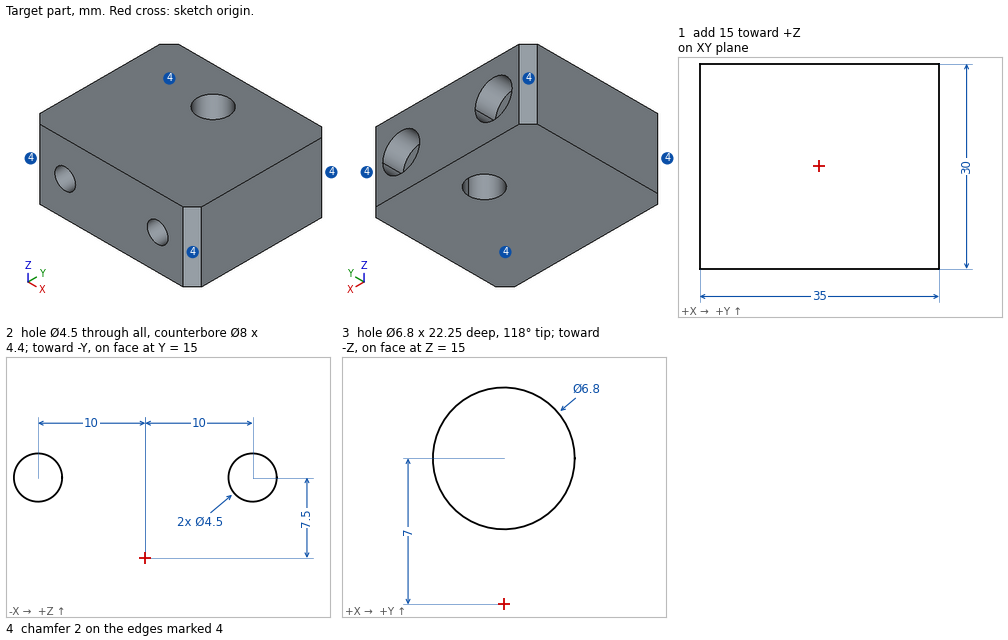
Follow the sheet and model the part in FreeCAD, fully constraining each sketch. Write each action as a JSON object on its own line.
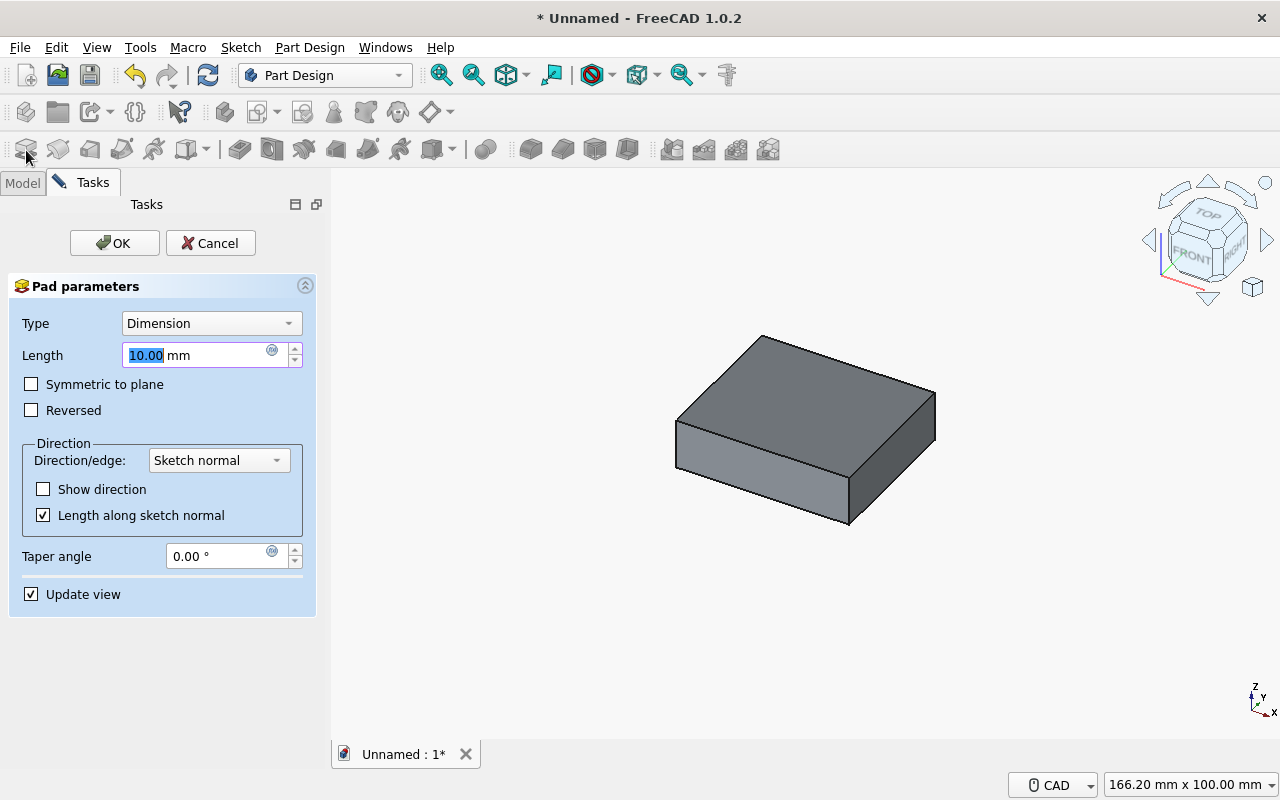
{"action": "type", "text": "15"}
{"action": "key", "text": "Tab"}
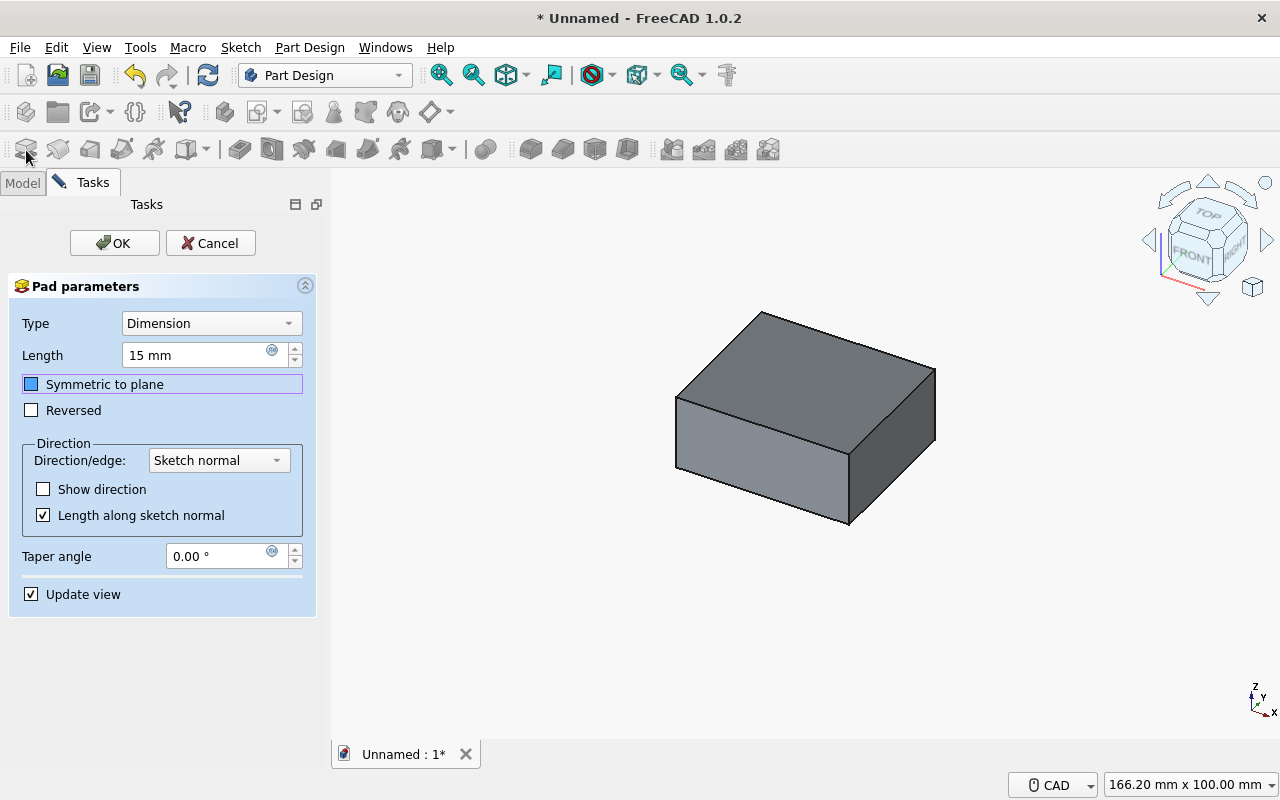
{"action": "left_click", "coordinate": [115, 243]}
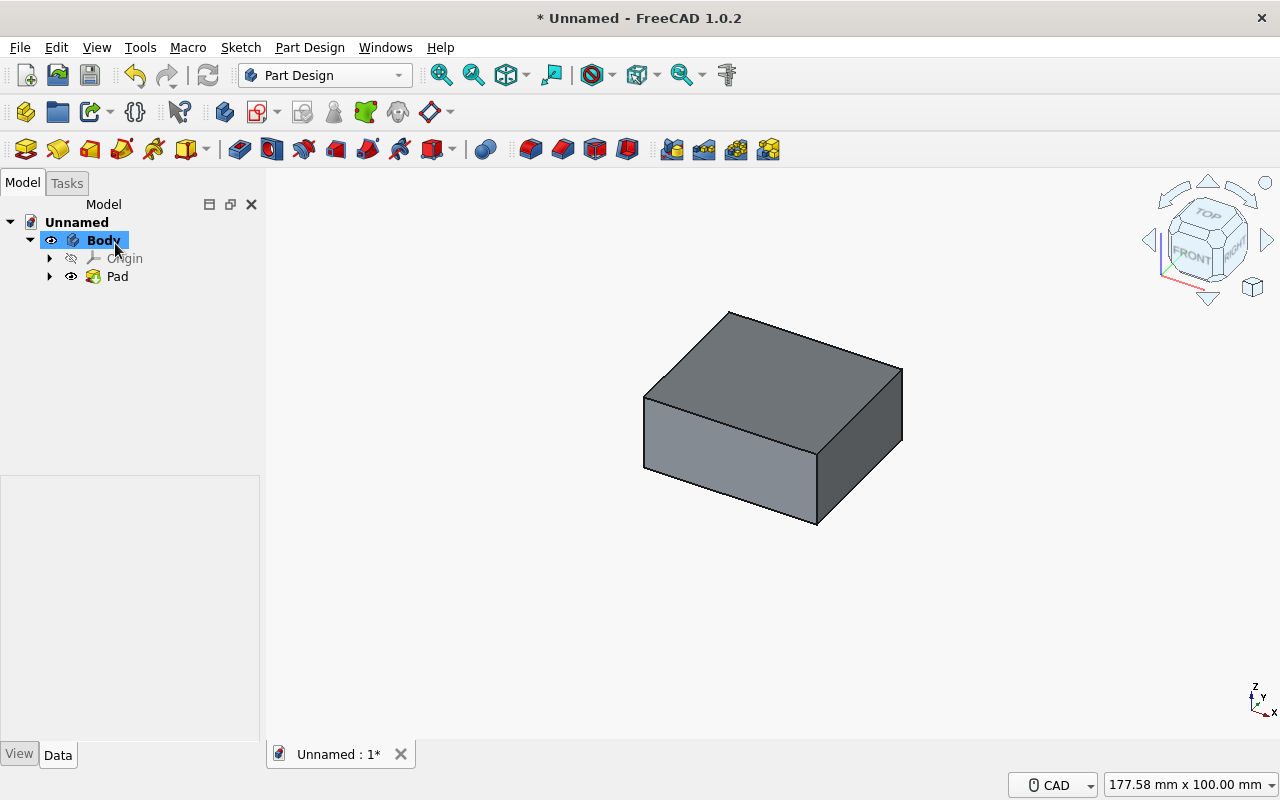
{"action": "left_click", "coordinate": [442, 76]}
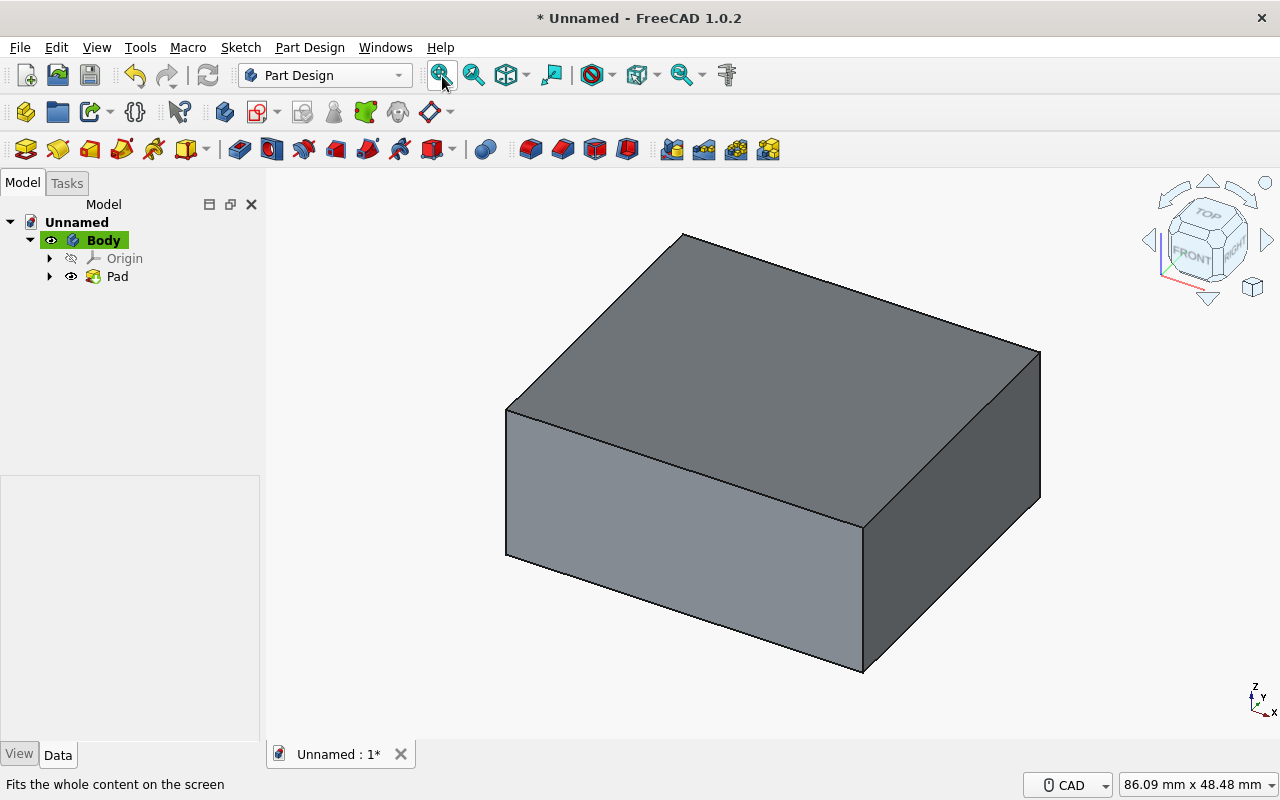
{"action": "key", "text": "4"}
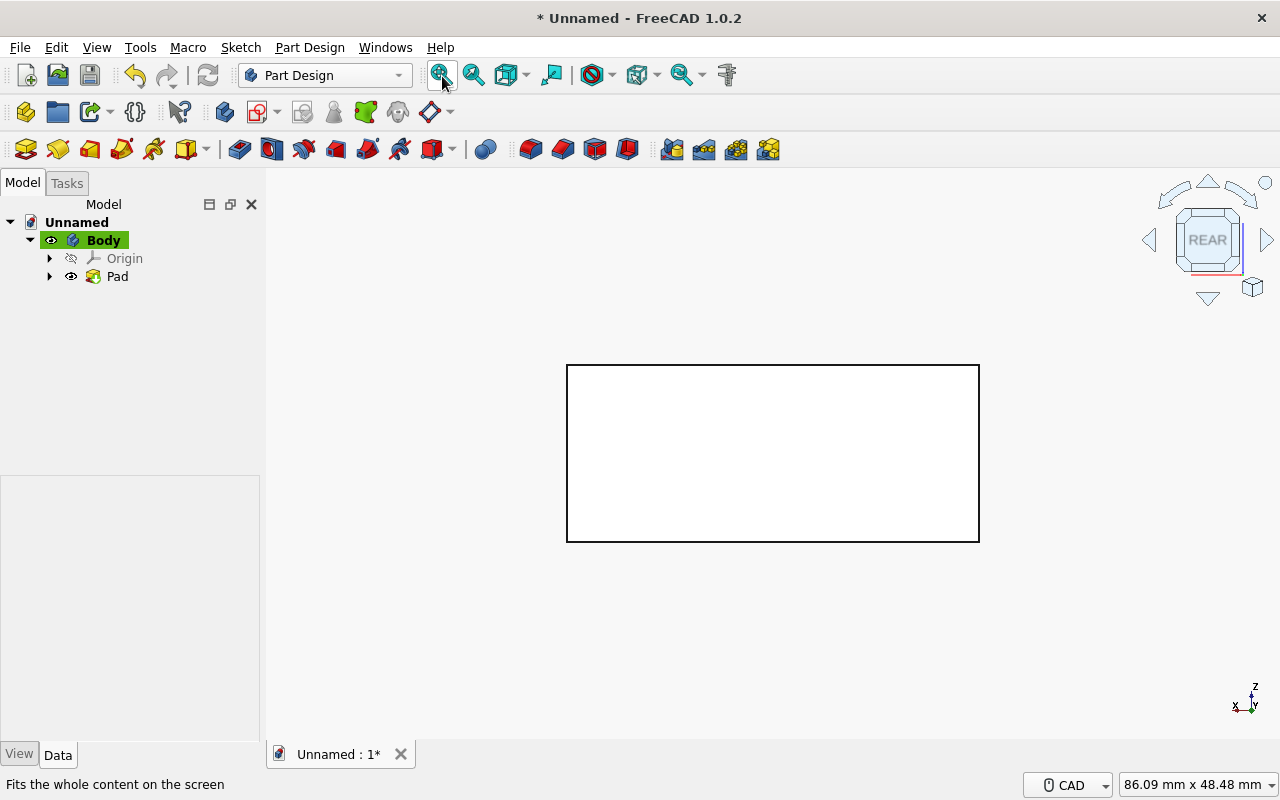
{"action": "key", "text": "v f"}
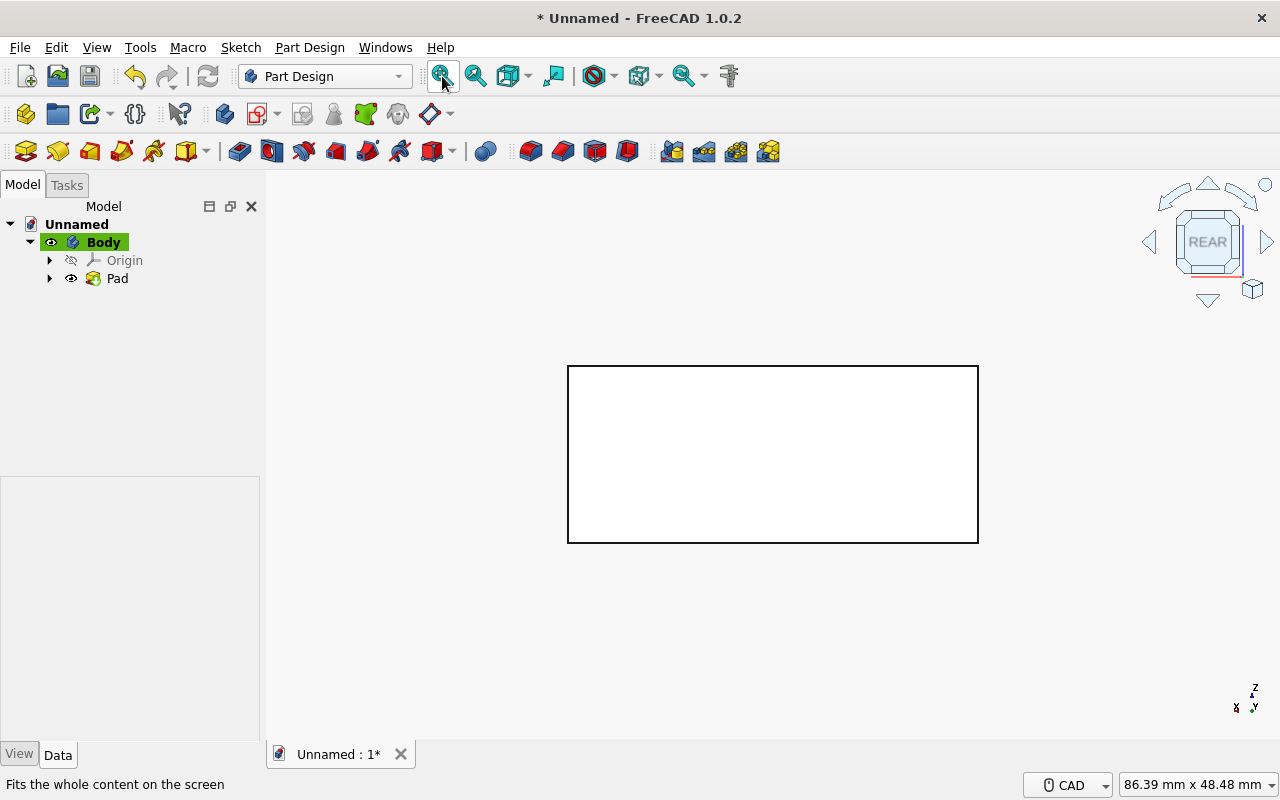
{"action": "left_click", "coordinate": [656, 454]}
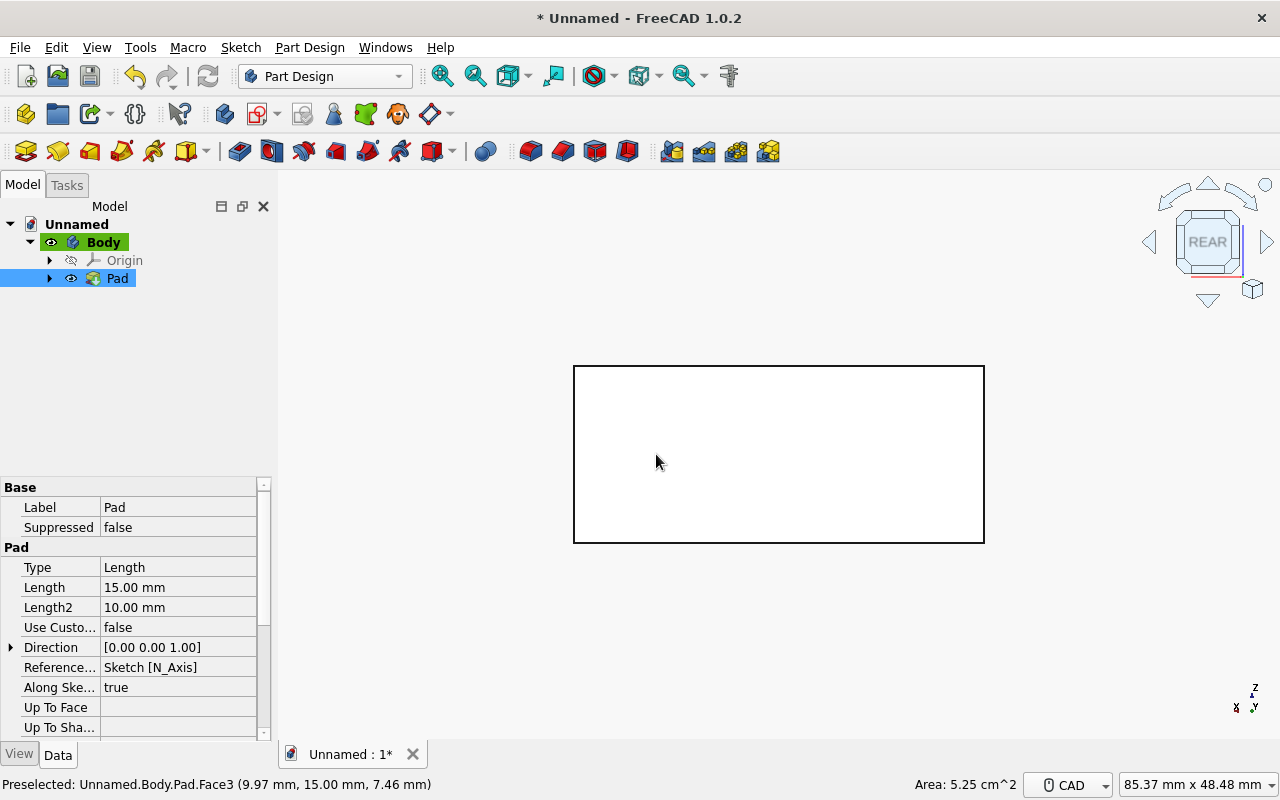
{"action": "left_click", "coordinate": [258, 114]}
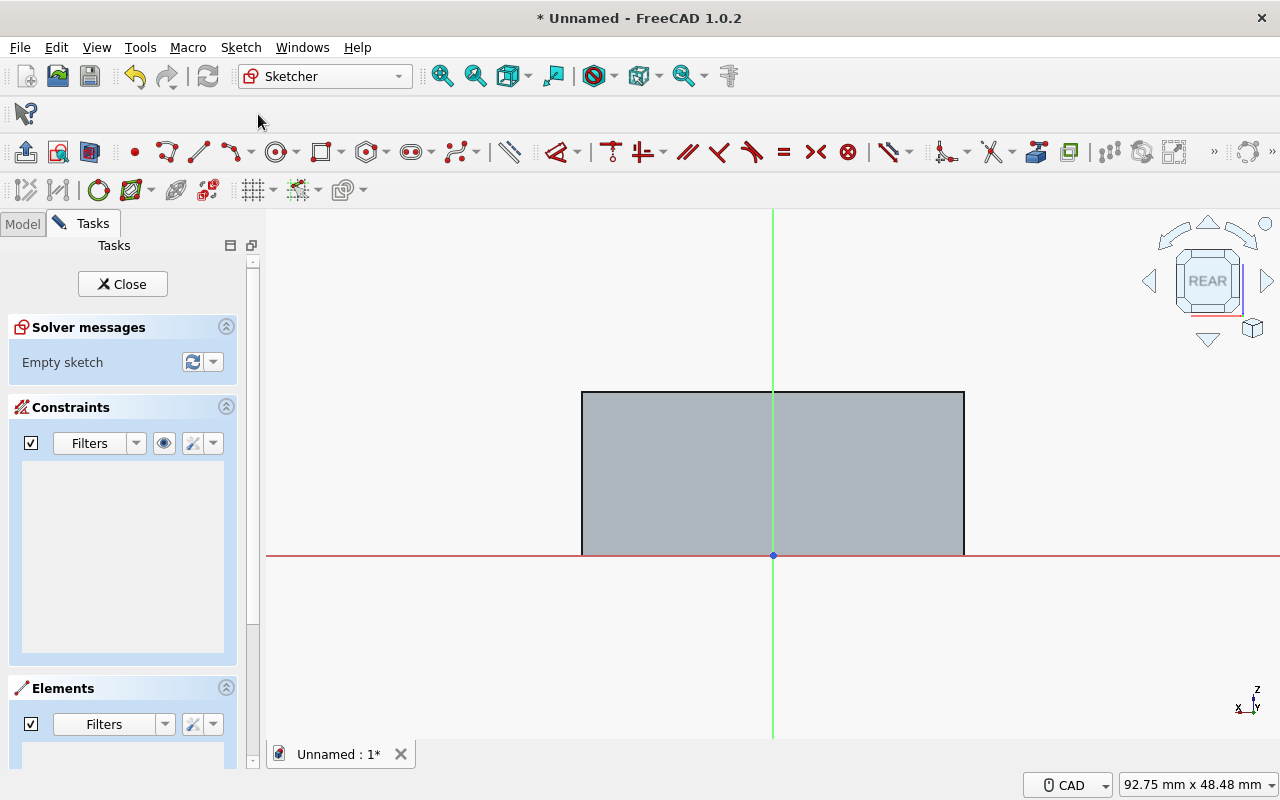
{"action": "scroll", "coordinate": [829, 526], "scroll_direction": "up", "scroll_amount": 4}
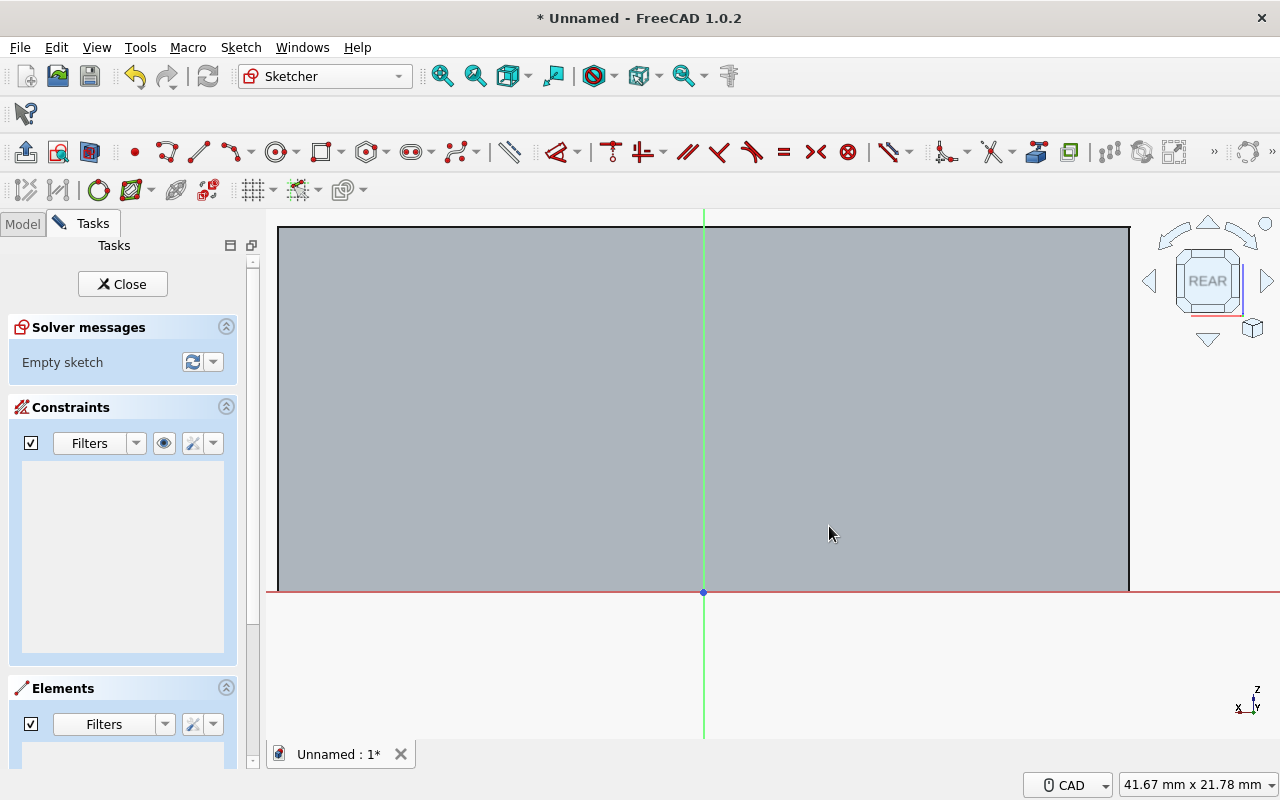
{"action": "left_click", "coordinate": [276, 152]}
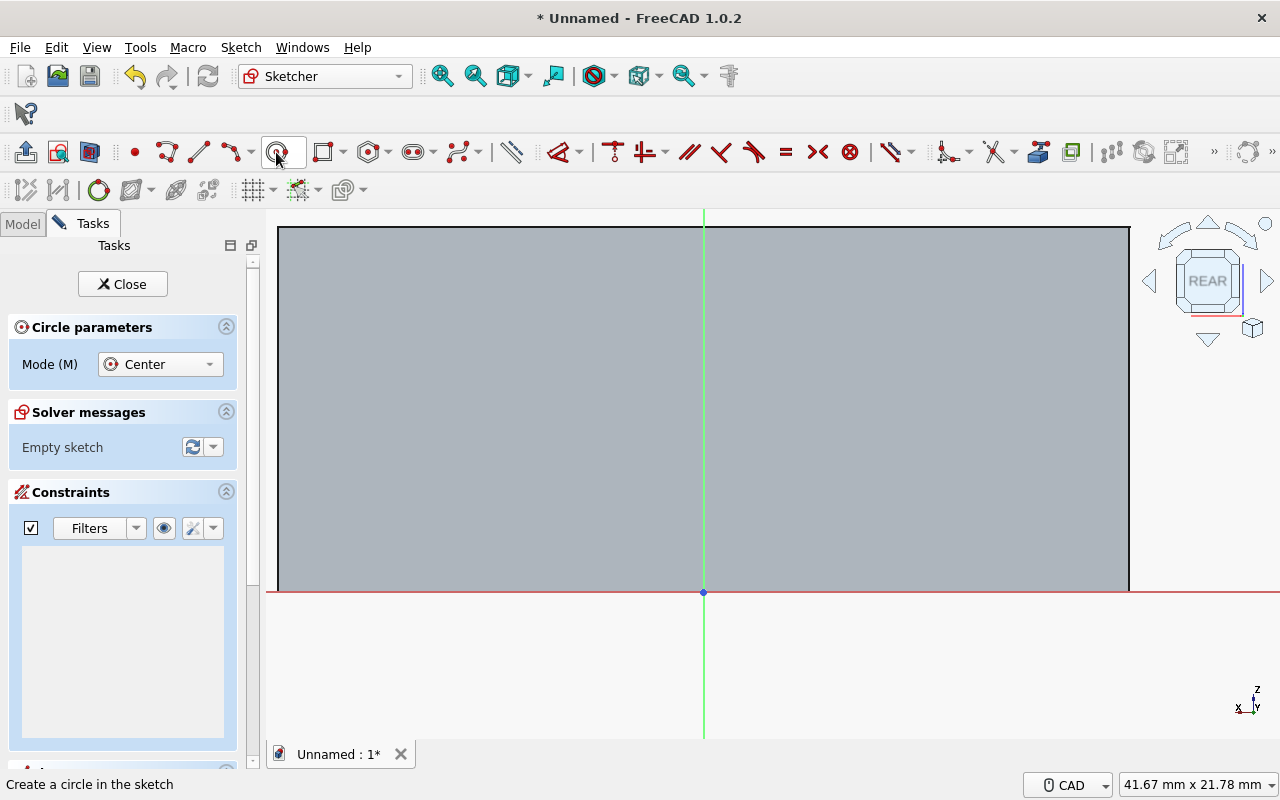
{"action": "left_click", "coordinate": [947, 410]}
{"action": "mouse_move", "coordinate": [986, 371]}